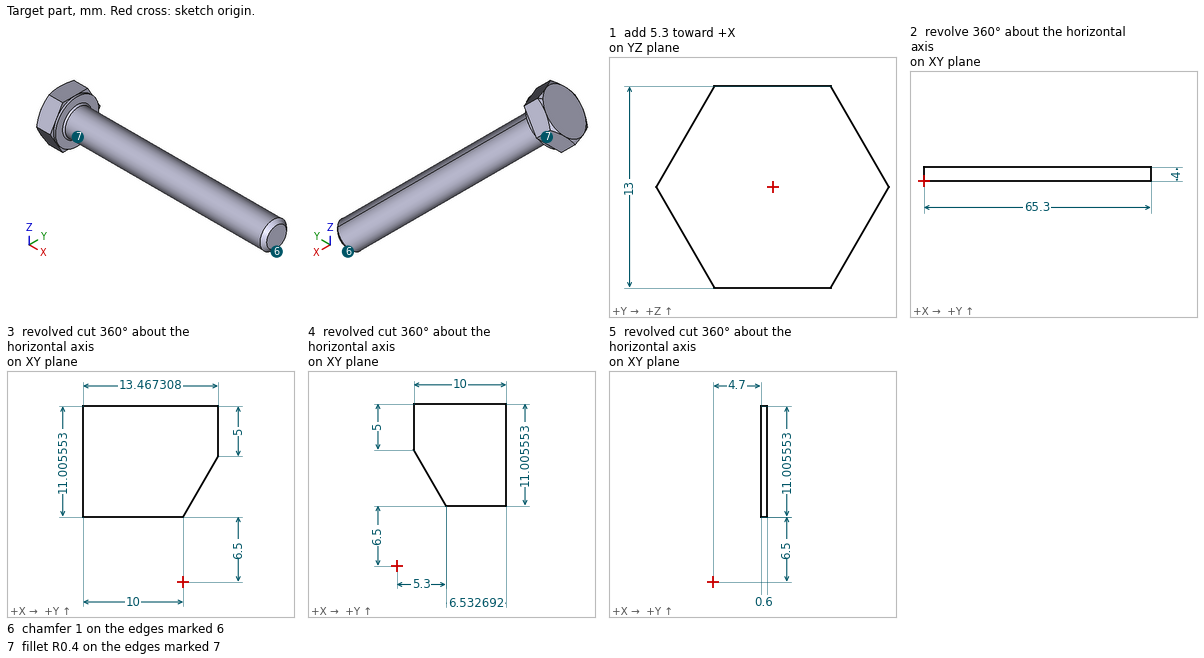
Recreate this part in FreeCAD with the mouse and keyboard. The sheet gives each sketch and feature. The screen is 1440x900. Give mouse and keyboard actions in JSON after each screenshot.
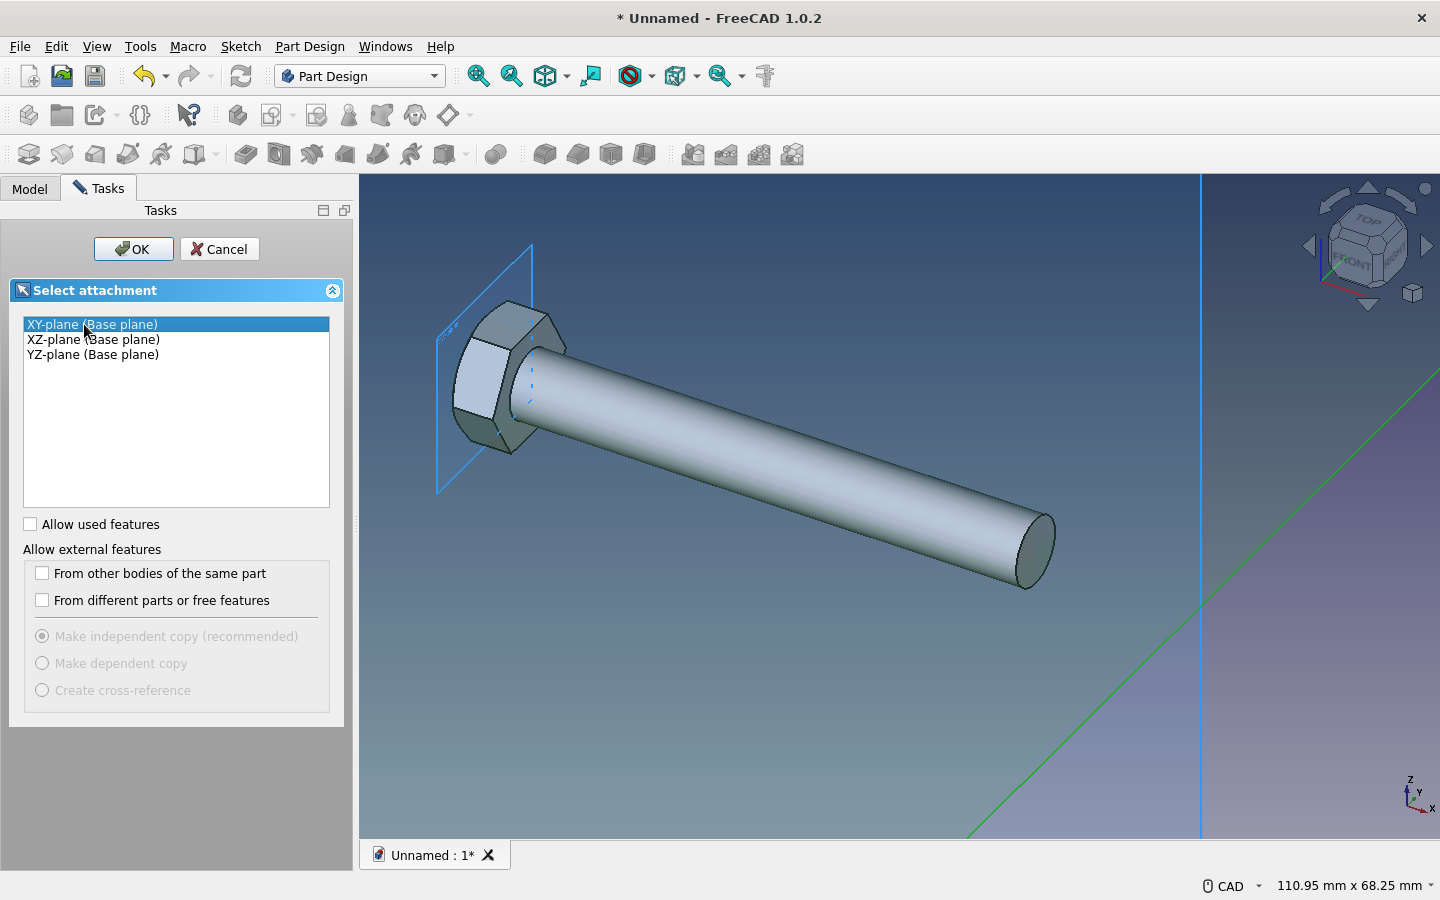
{"action": "left_click", "coordinate": [134, 249]}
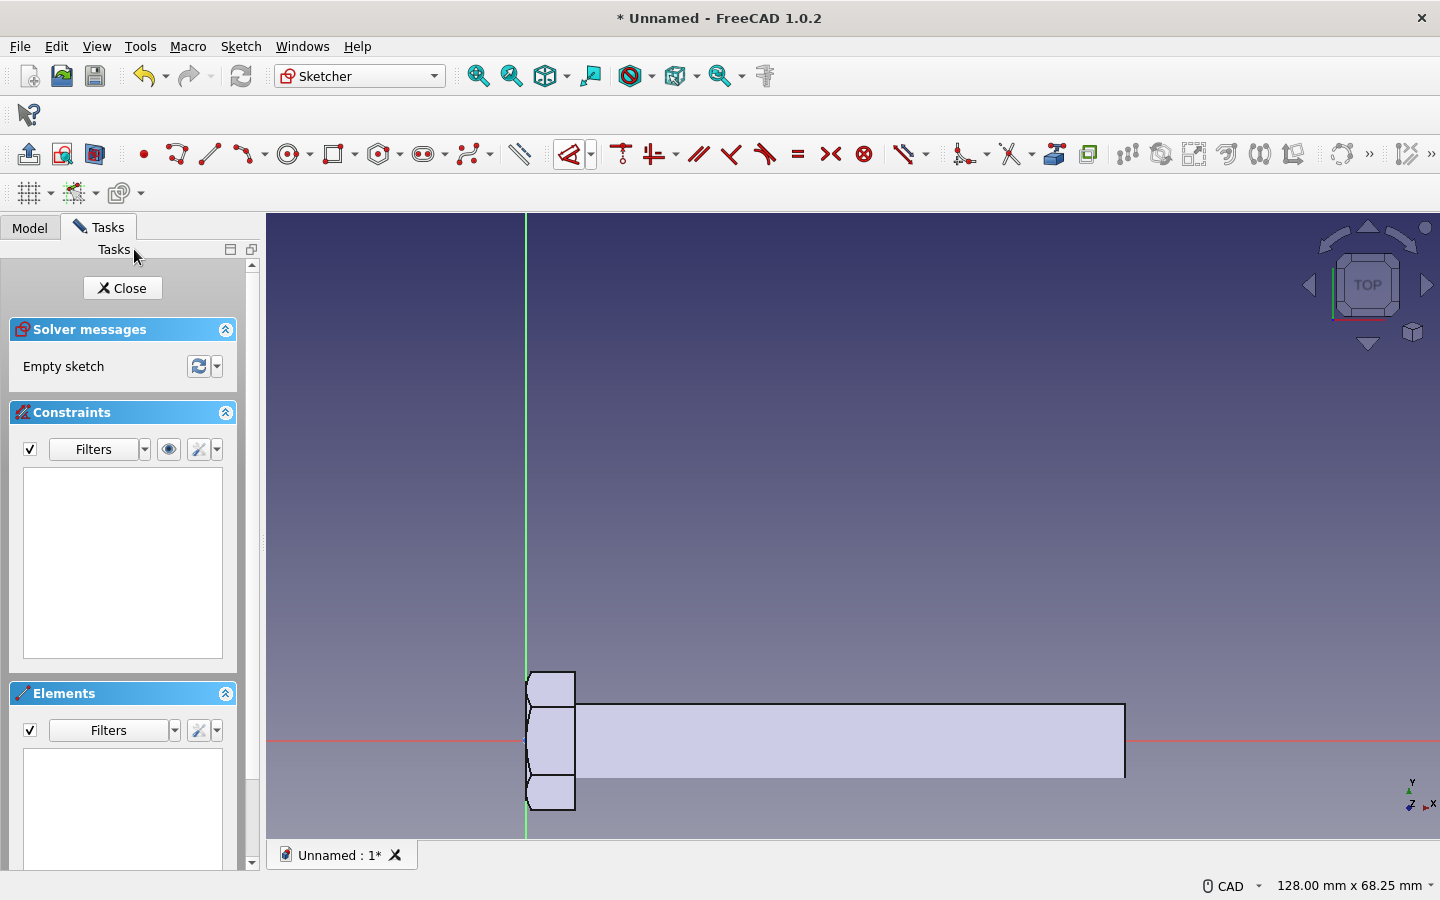
{"action": "left_click", "coordinate": [95, 154]}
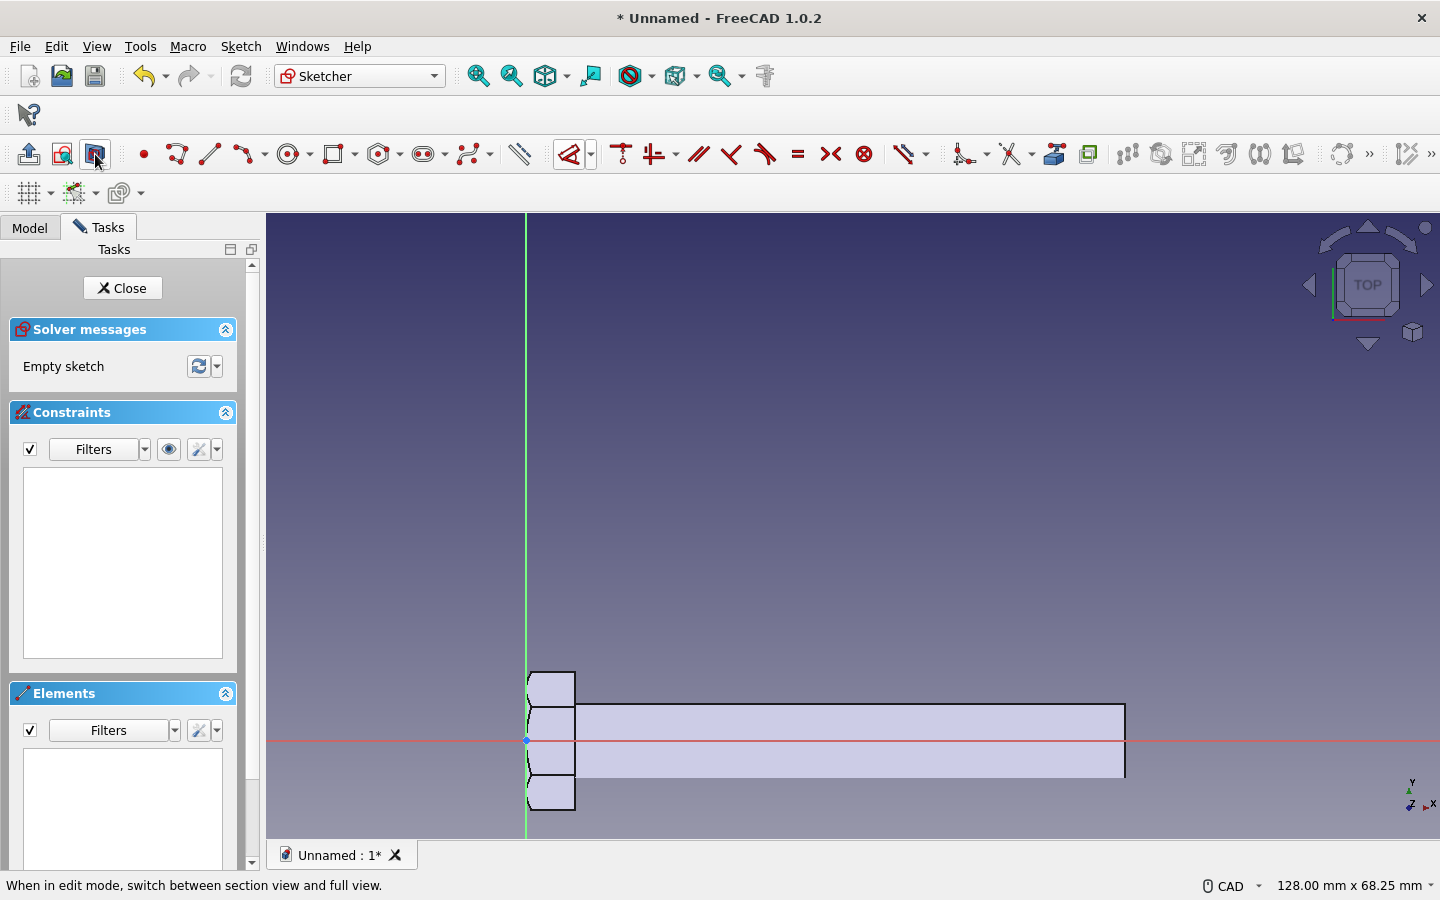
{"action": "scroll", "coordinate": [462, 739], "scroll_direction": "up", "scroll_amount": 5}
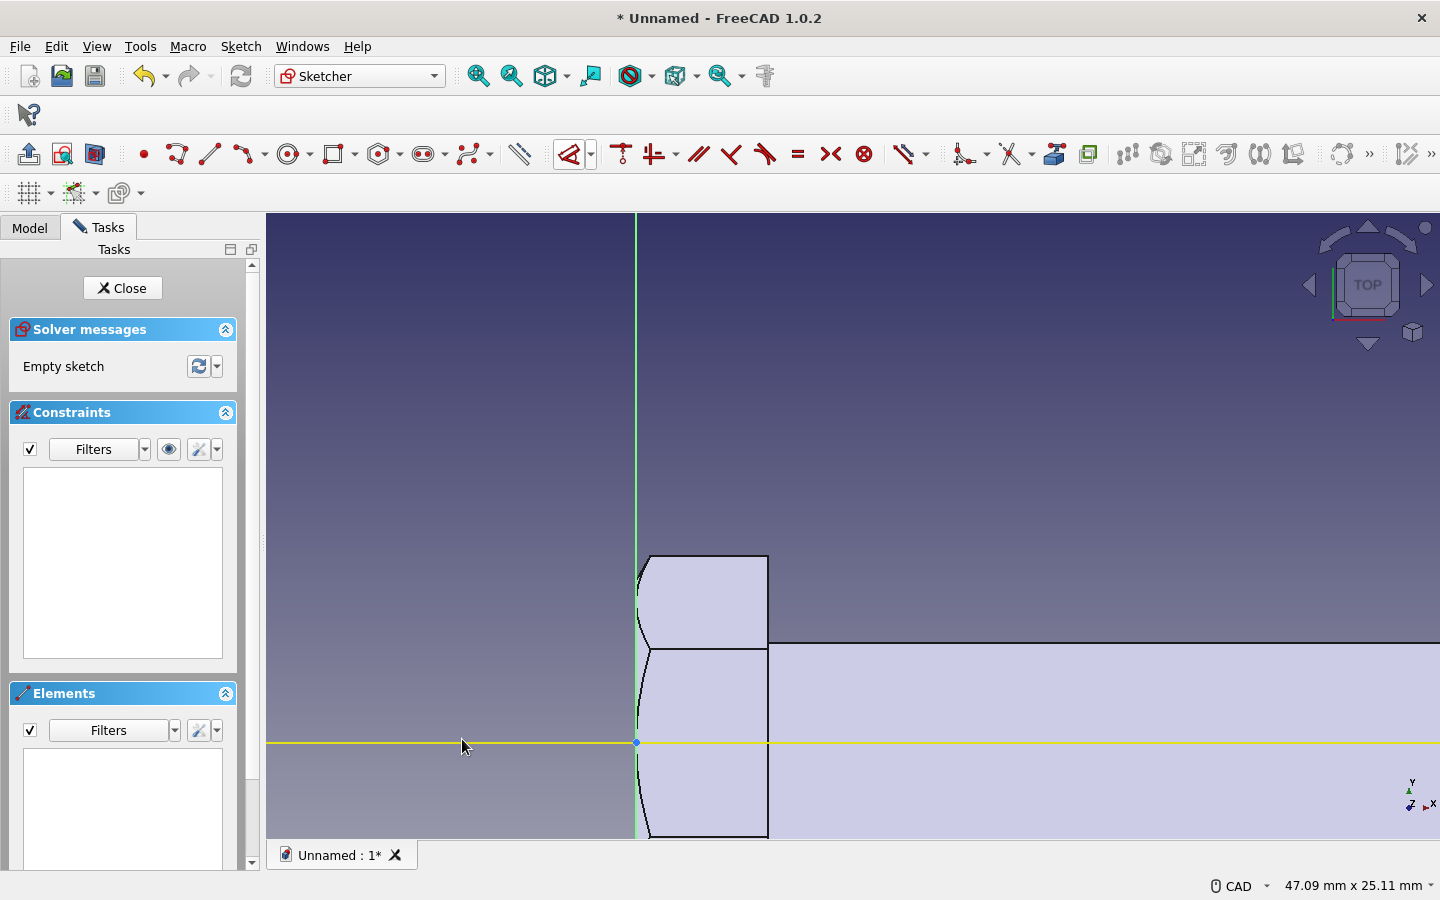
{"action": "left_click", "coordinate": [177, 154]}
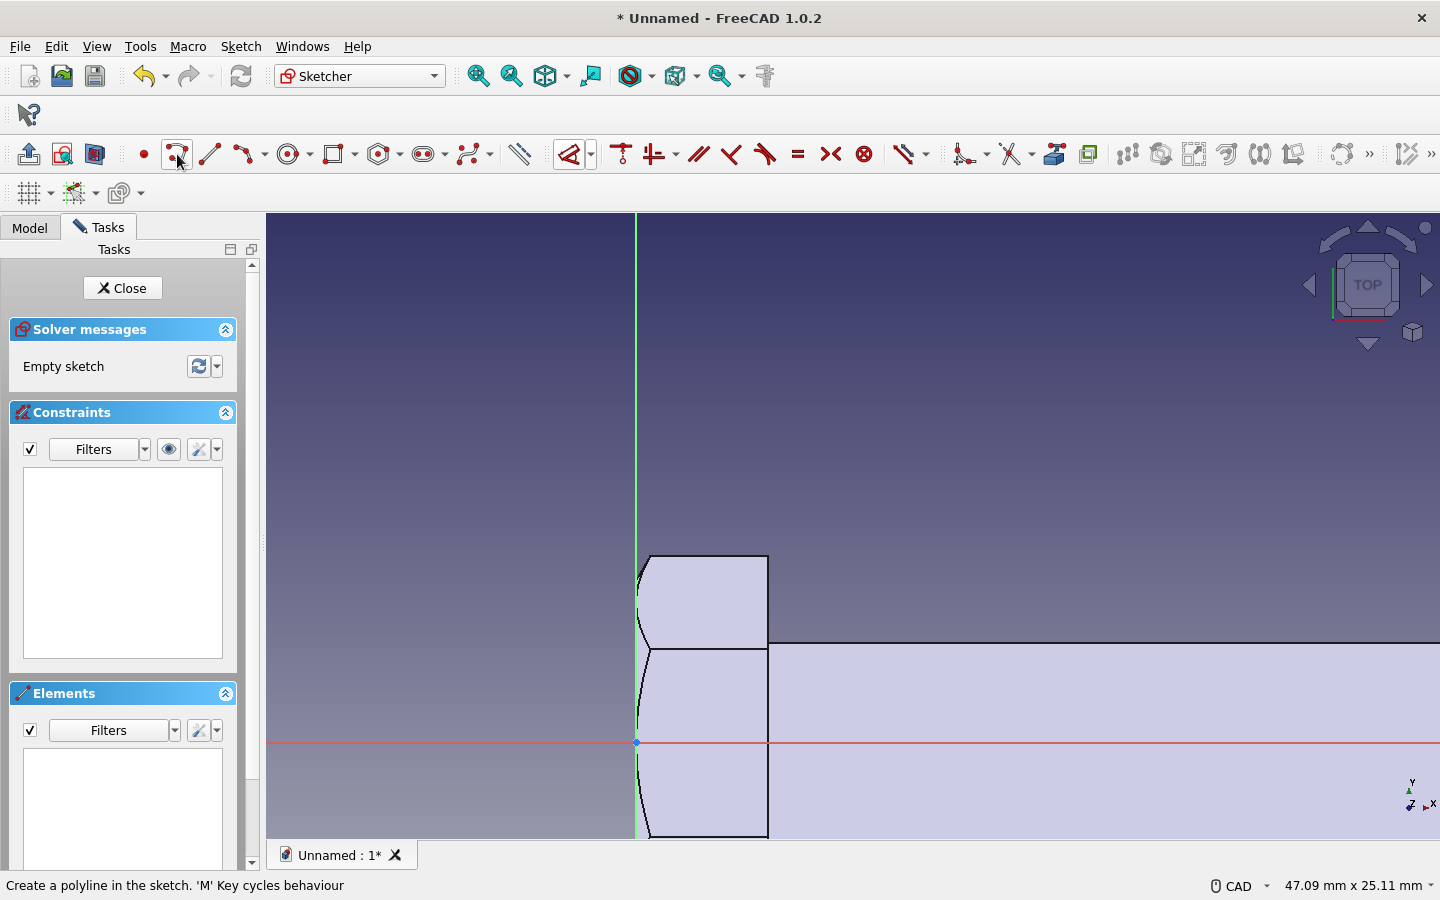
{"action": "left_click", "coordinate": [768, 581]}
{"action": "left_click", "coordinate": [931, 581]}
{"action": "left_click", "coordinate": [931, 307]}
{"action": "left_click", "coordinate": [682, 307]}
{"action": "left_click", "coordinate": [682, 431]}
{"action": "left_click", "coordinate": [768, 582]}
{"action": "key", "text": "Escape"}
{"action": "key", "text": "Escape"}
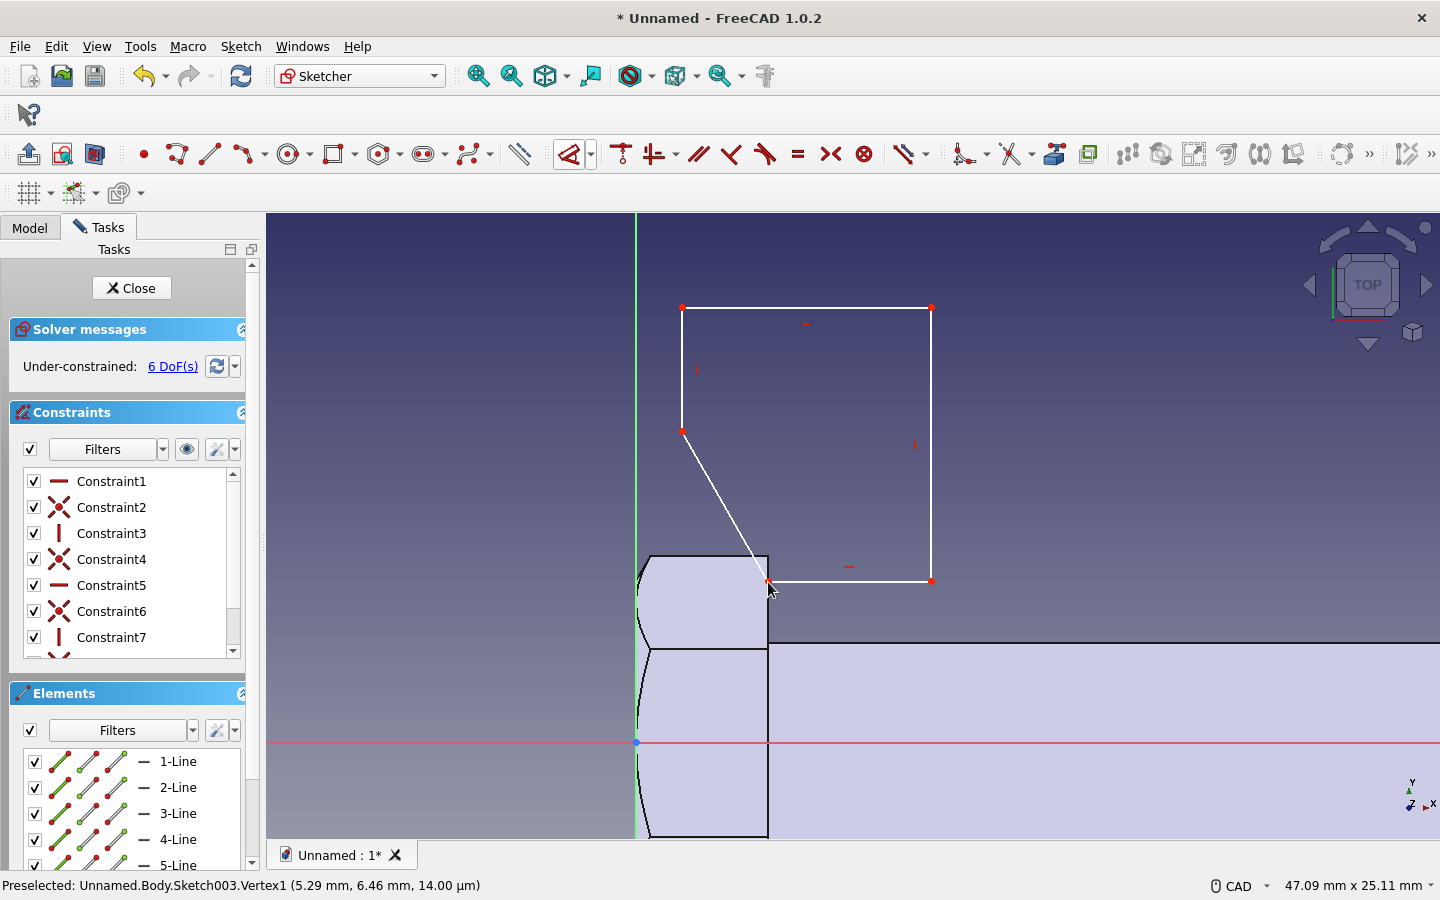
{"action": "left_click", "coordinate": [682, 345]}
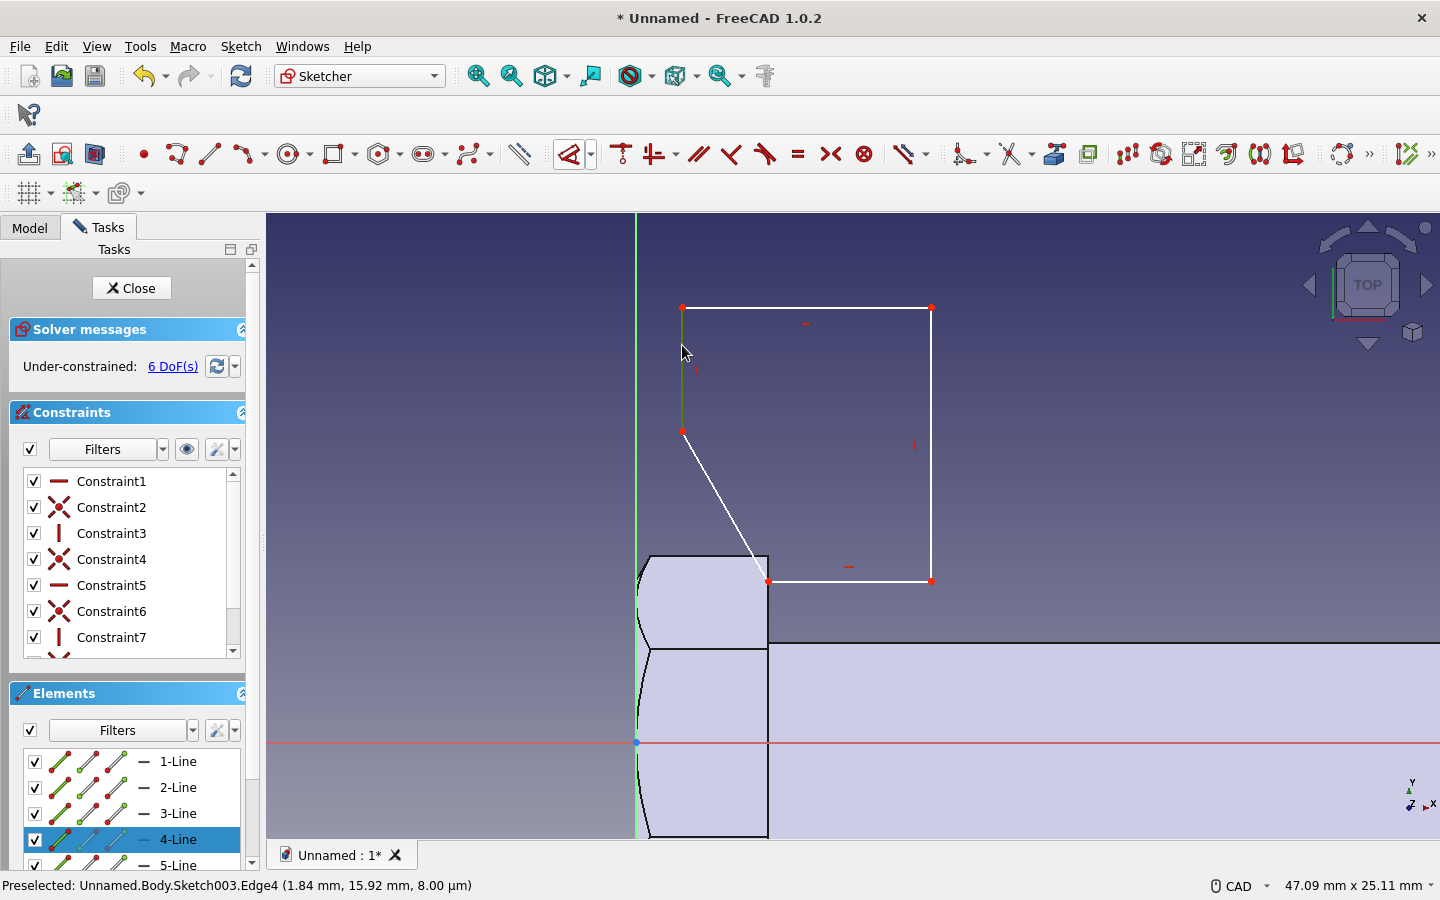
{"action": "key", "text": "i"}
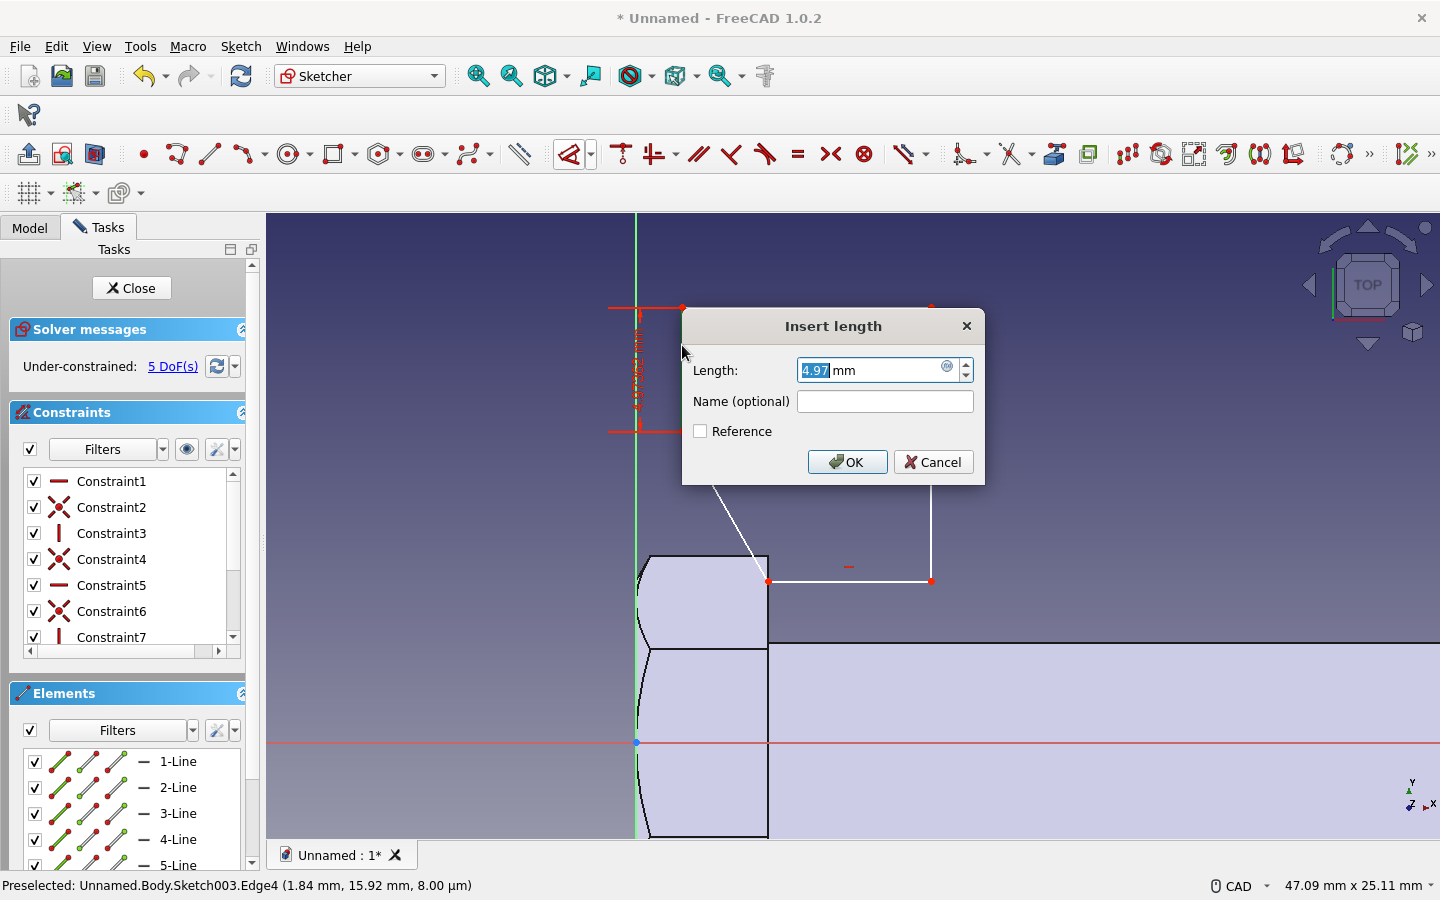
{"action": "type", "text": "5"}
{"action": "key", "text": "Return"}